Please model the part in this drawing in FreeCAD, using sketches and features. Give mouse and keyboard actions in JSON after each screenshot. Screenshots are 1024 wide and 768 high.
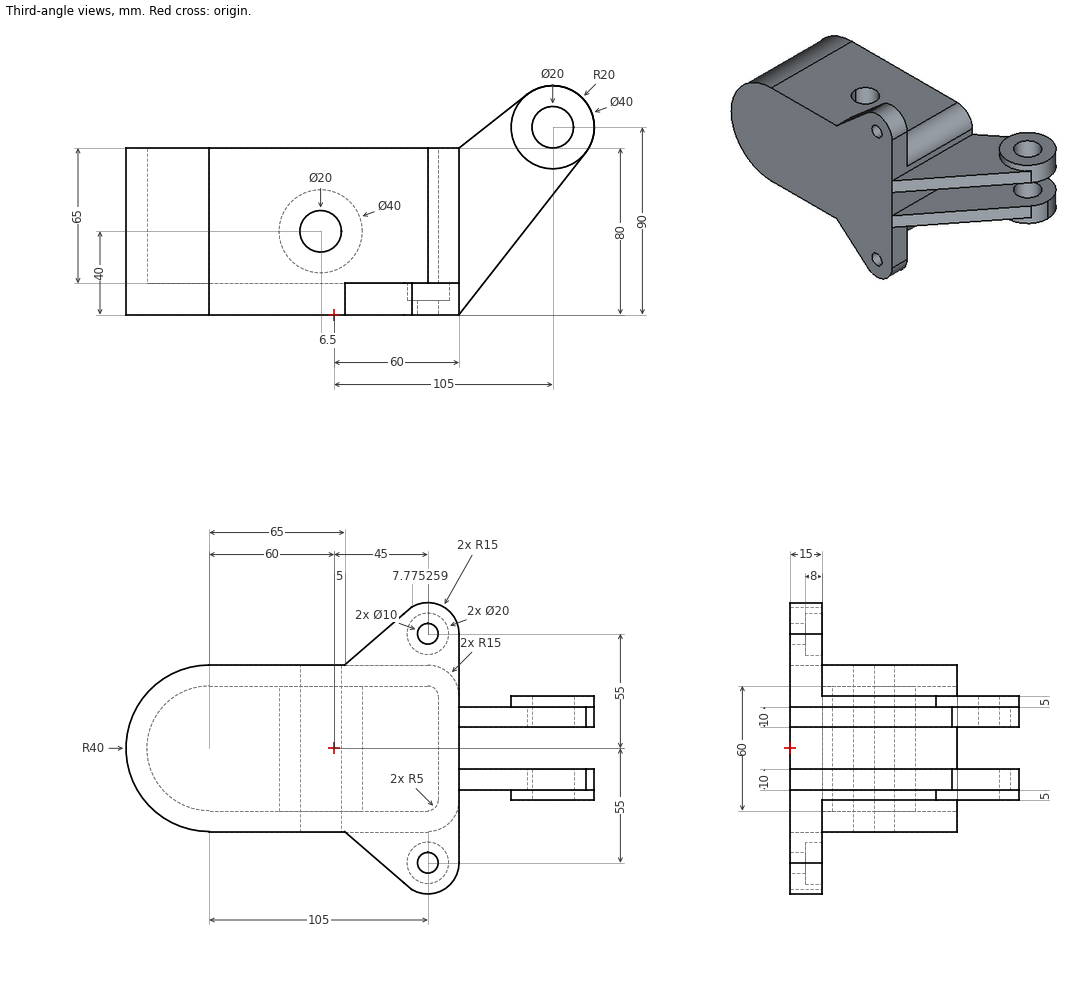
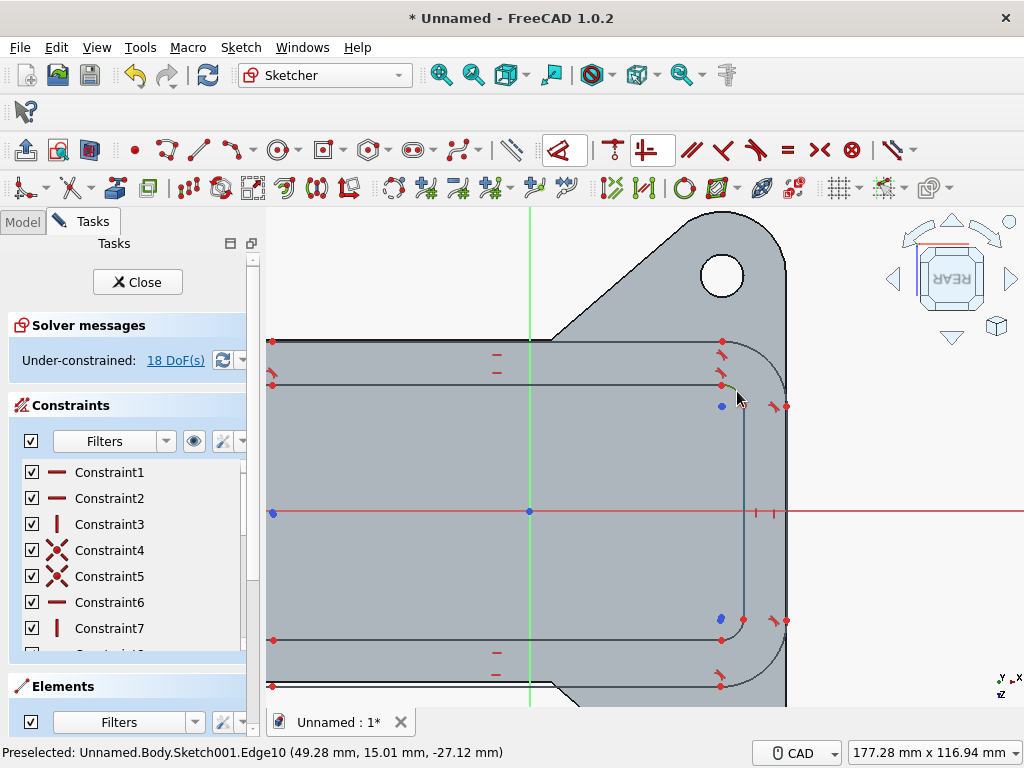
{"action": "left_click", "coordinate": [756, 150]}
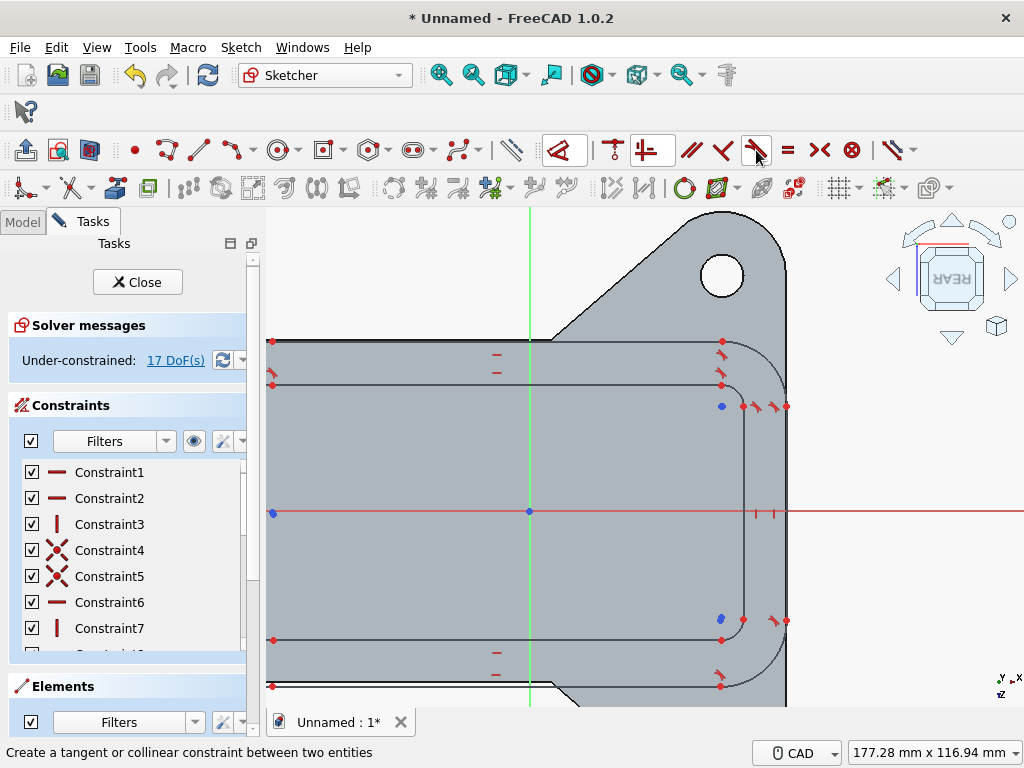
{"action": "left_click", "coordinate": [744, 471]}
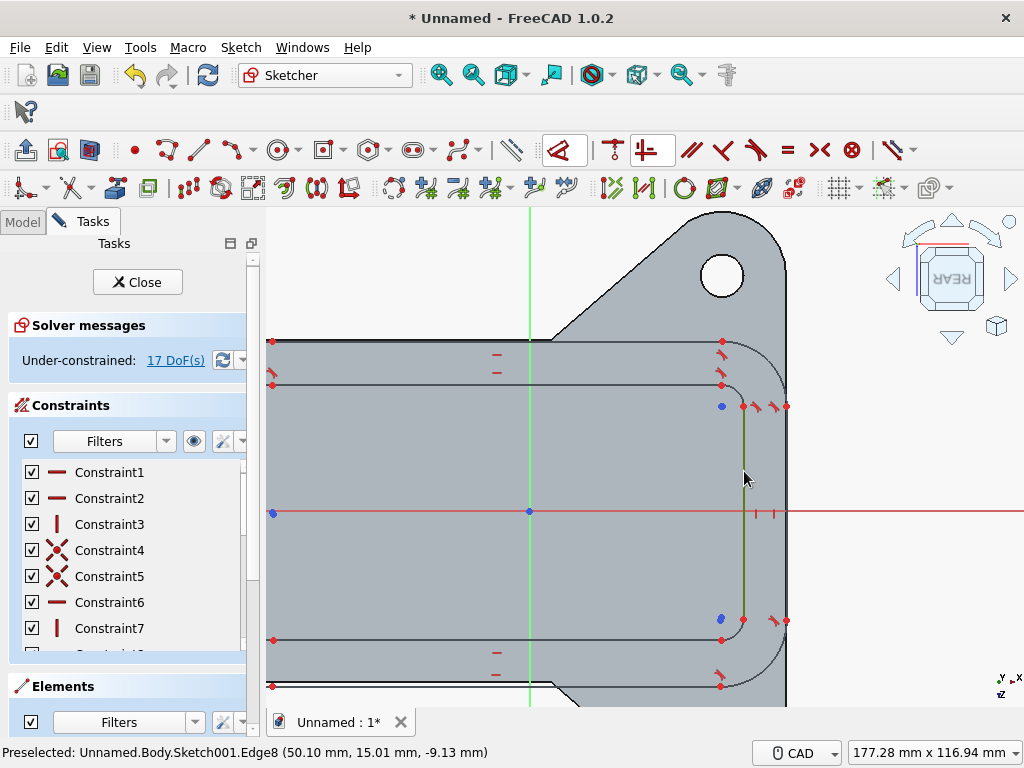
{"action": "scroll", "coordinate": [731, 638], "scroll_direction": "up", "scroll_amount": 2}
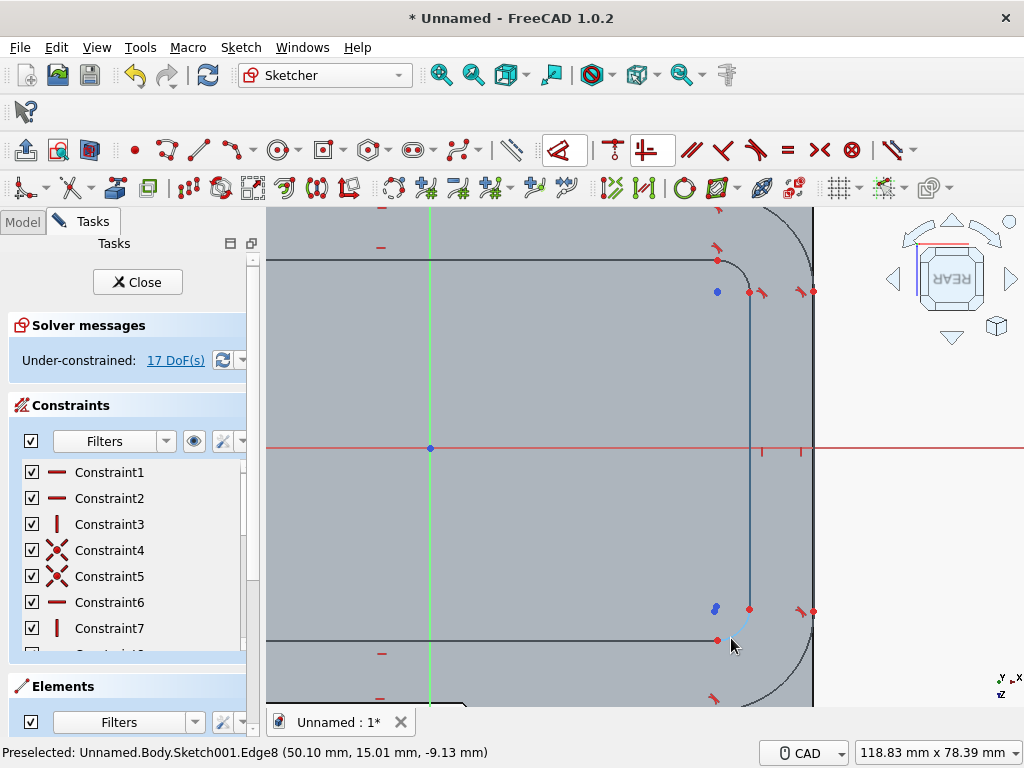
{"action": "left_click", "coordinate": [731, 637]}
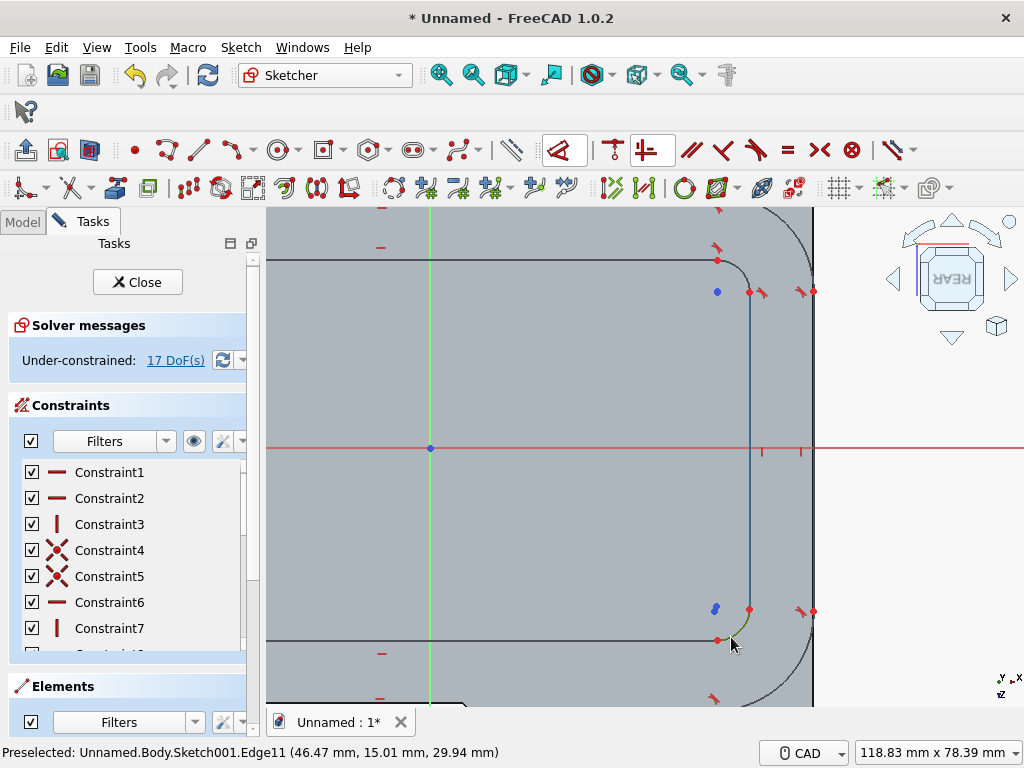
{"action": "left_click", "coordinate": [756, 150]}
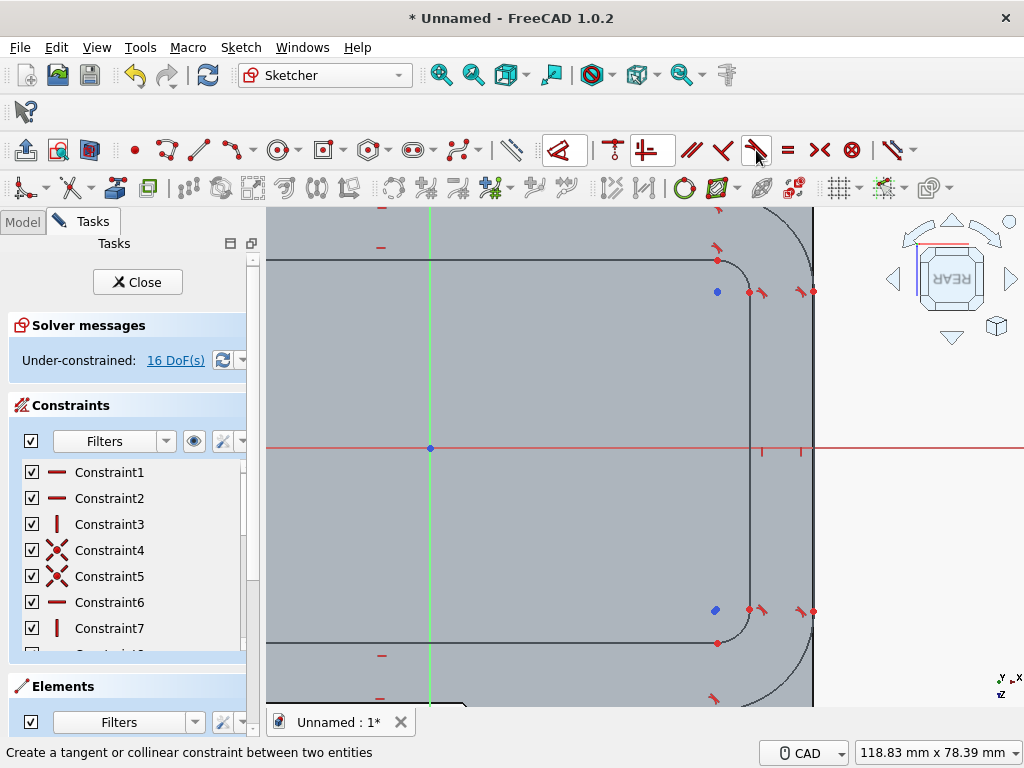
{"action": "left_click", "coordinate": [517, 643]}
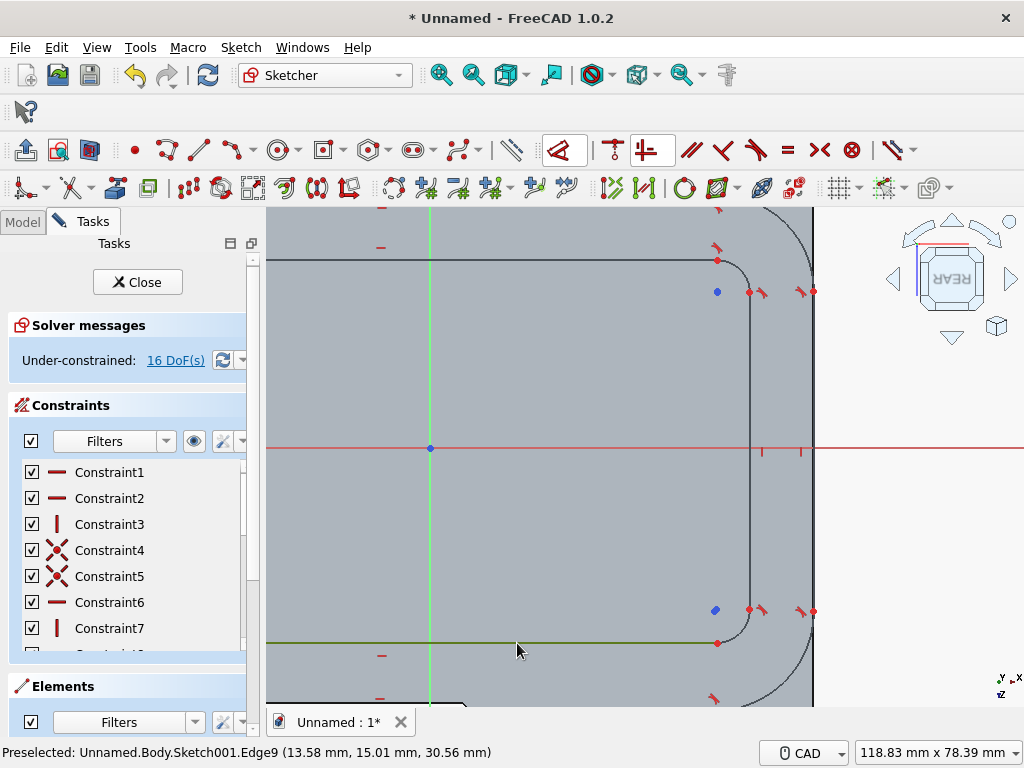
{"action": "left_click", "coordinate": [732, 639]}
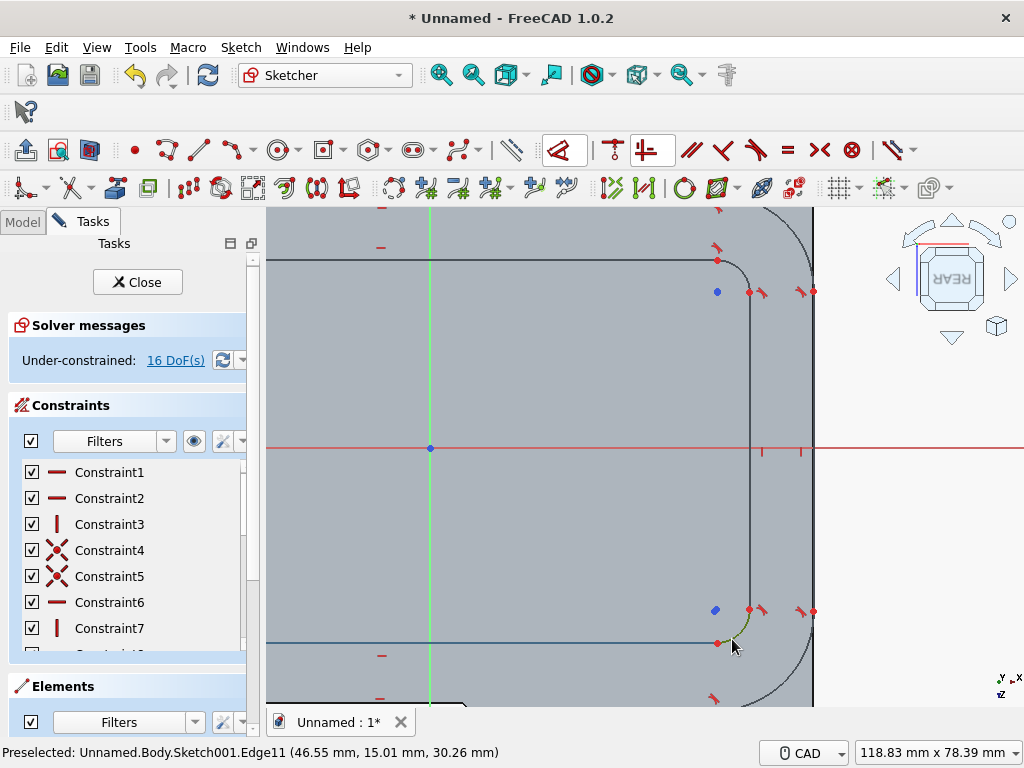
{"action": "left_click", "coordinate": [756, 150]}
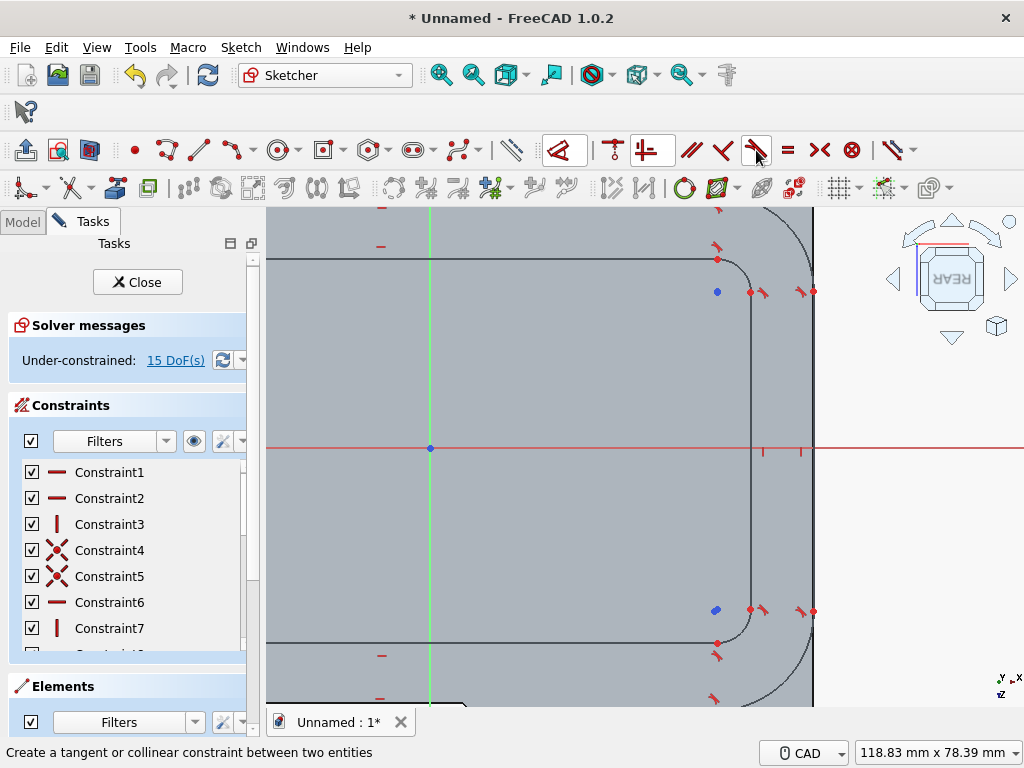
{"action": "left_click", "coordinate": [516, 643]}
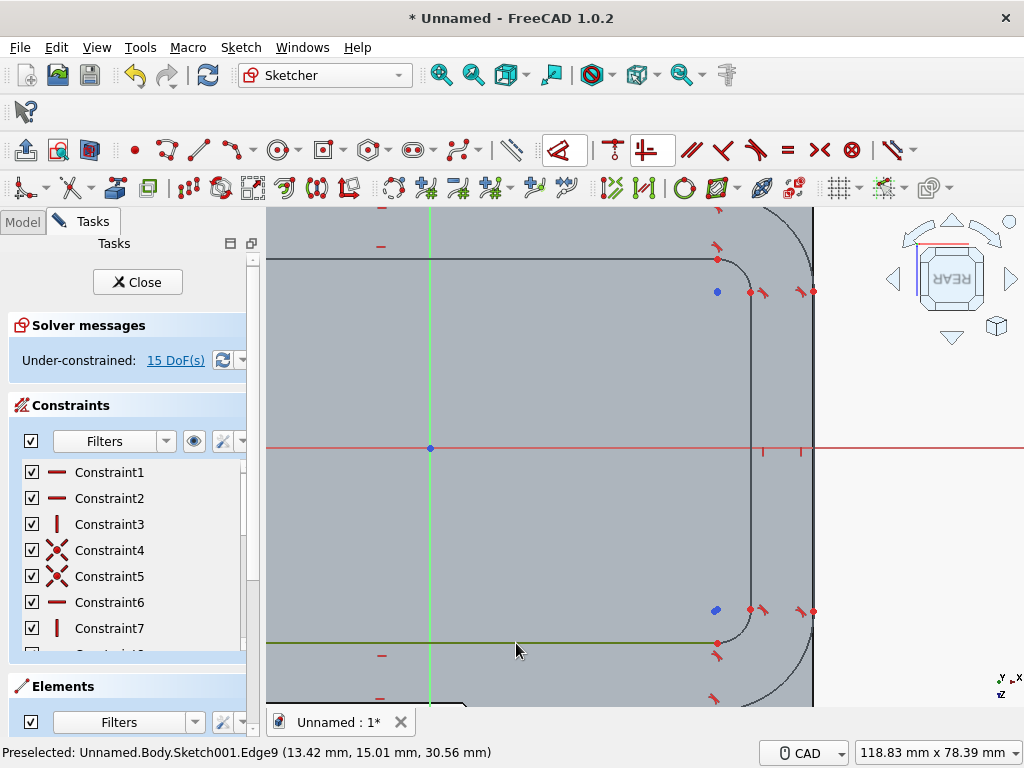
{"action": "scroll", "coordinate": [736, 462], "scroll_direction": "down", "scroll_amount": 5}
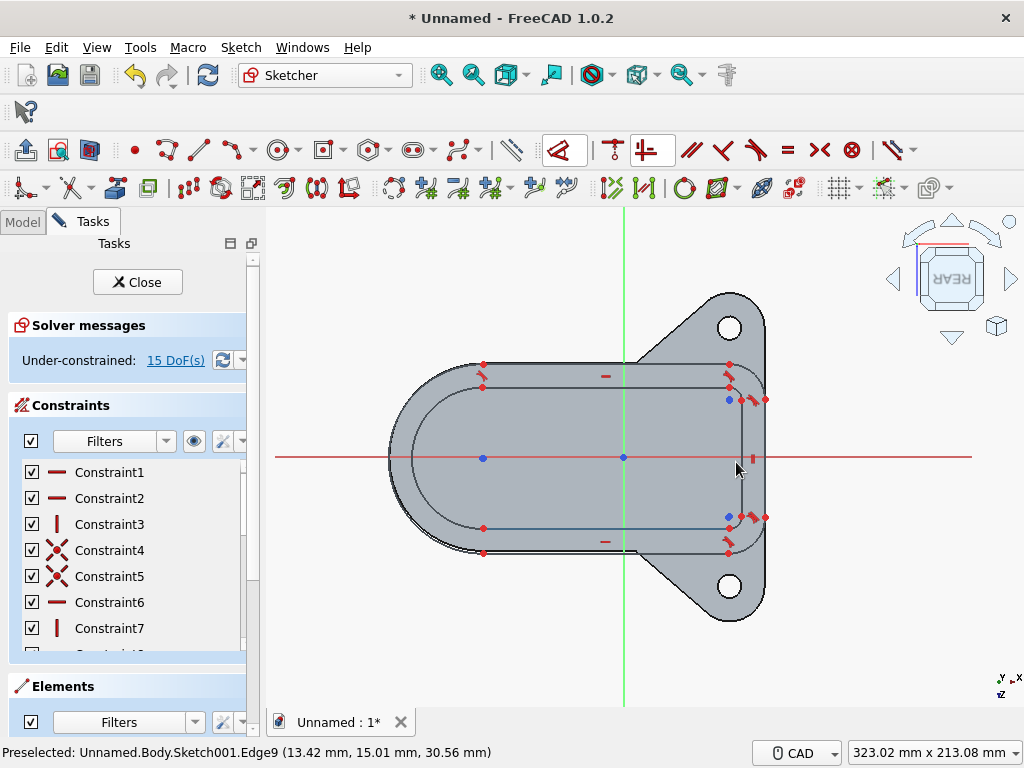
{"action": "left_click", "coordinate": [425, 417]}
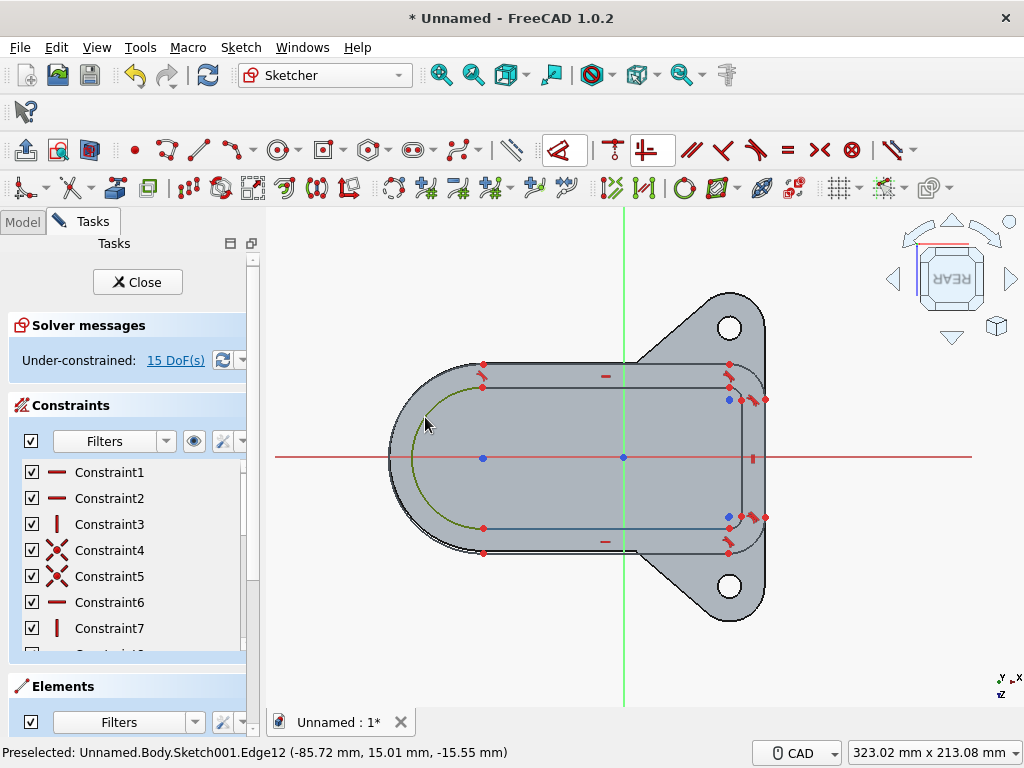
{"action": "left_click", "coordinate": [756, 150]}